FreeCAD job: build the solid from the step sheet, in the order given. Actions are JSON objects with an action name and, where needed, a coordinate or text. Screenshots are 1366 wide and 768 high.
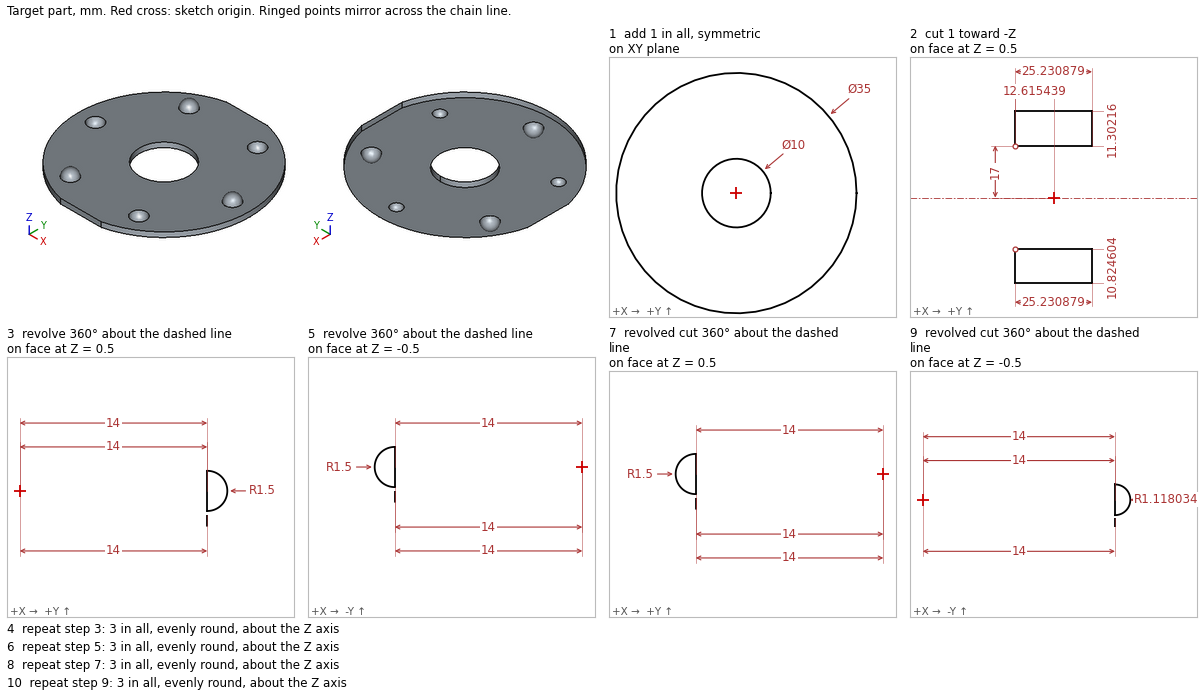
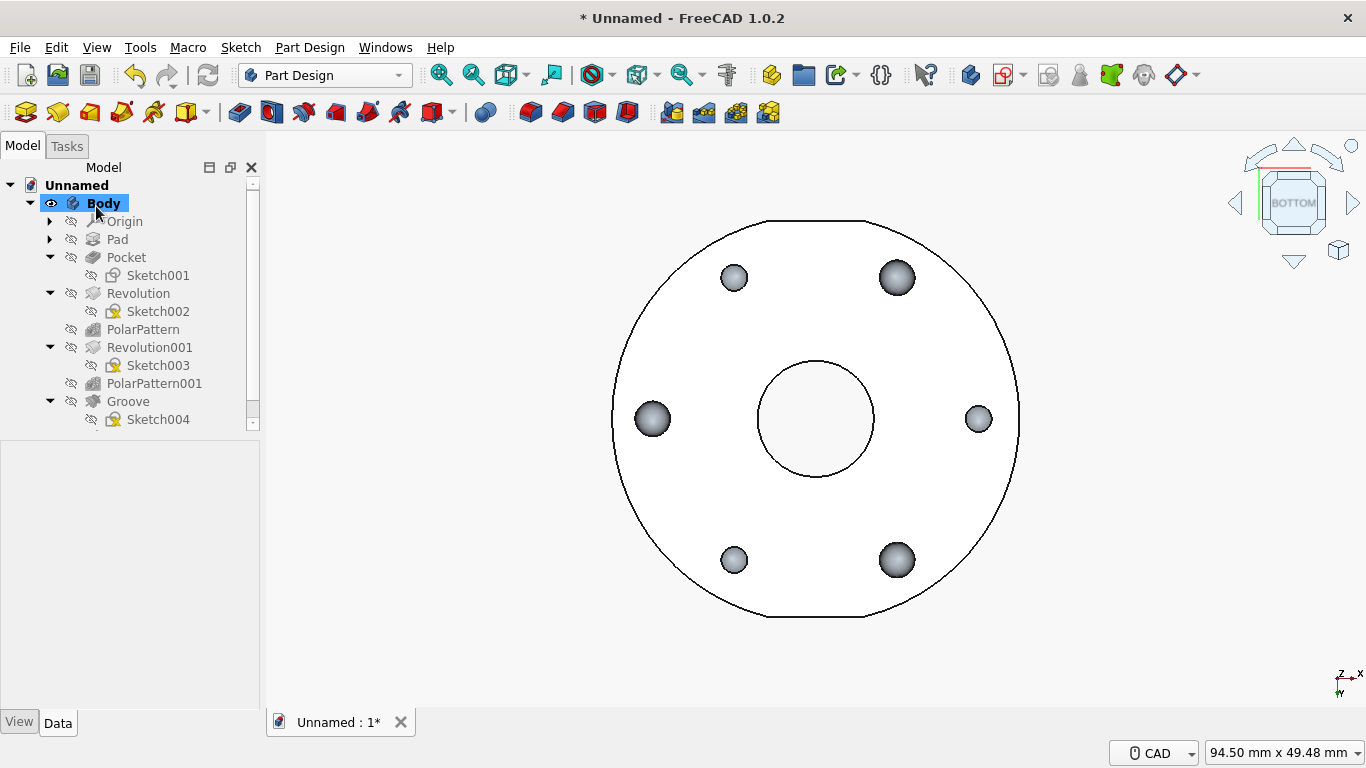
{"action": "left_click", "coordinate": [932, 361]}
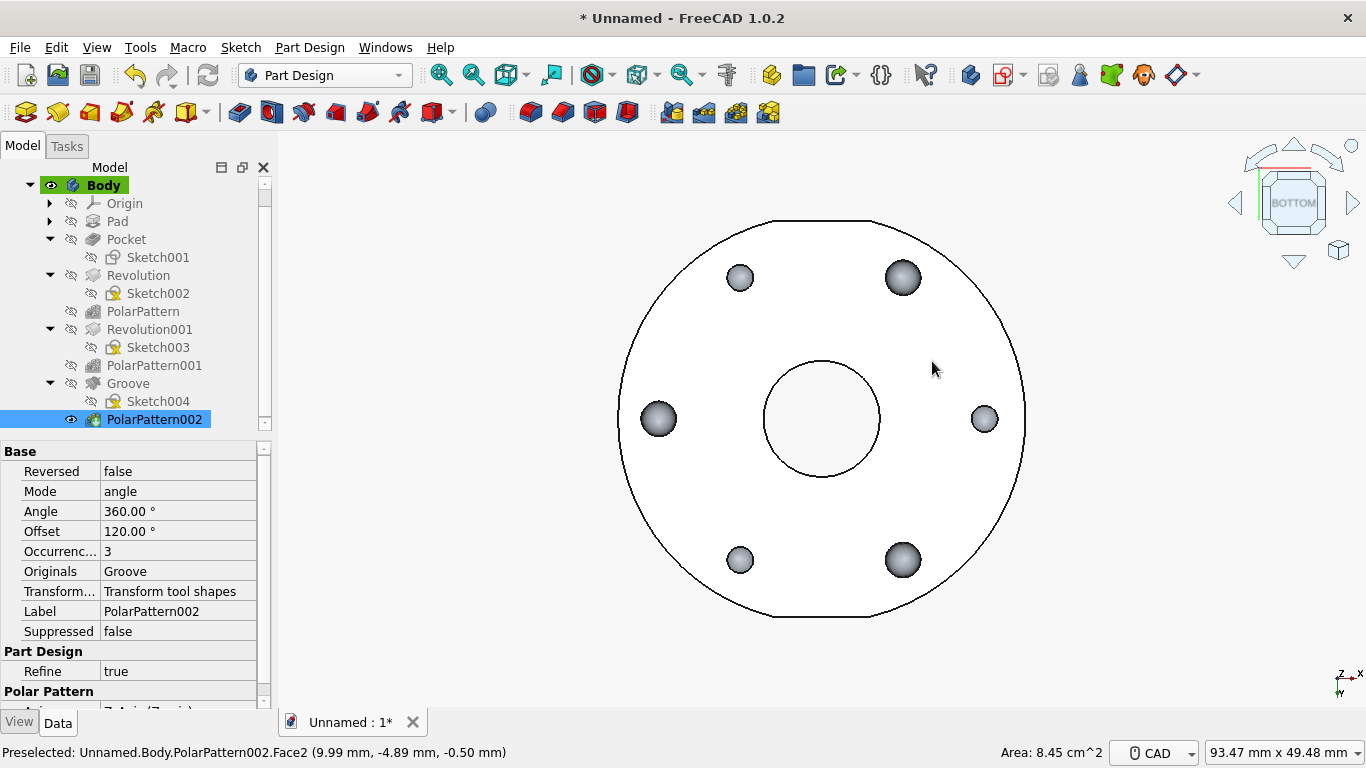
{"action": "left_click", "coordinate": [1004, 76]}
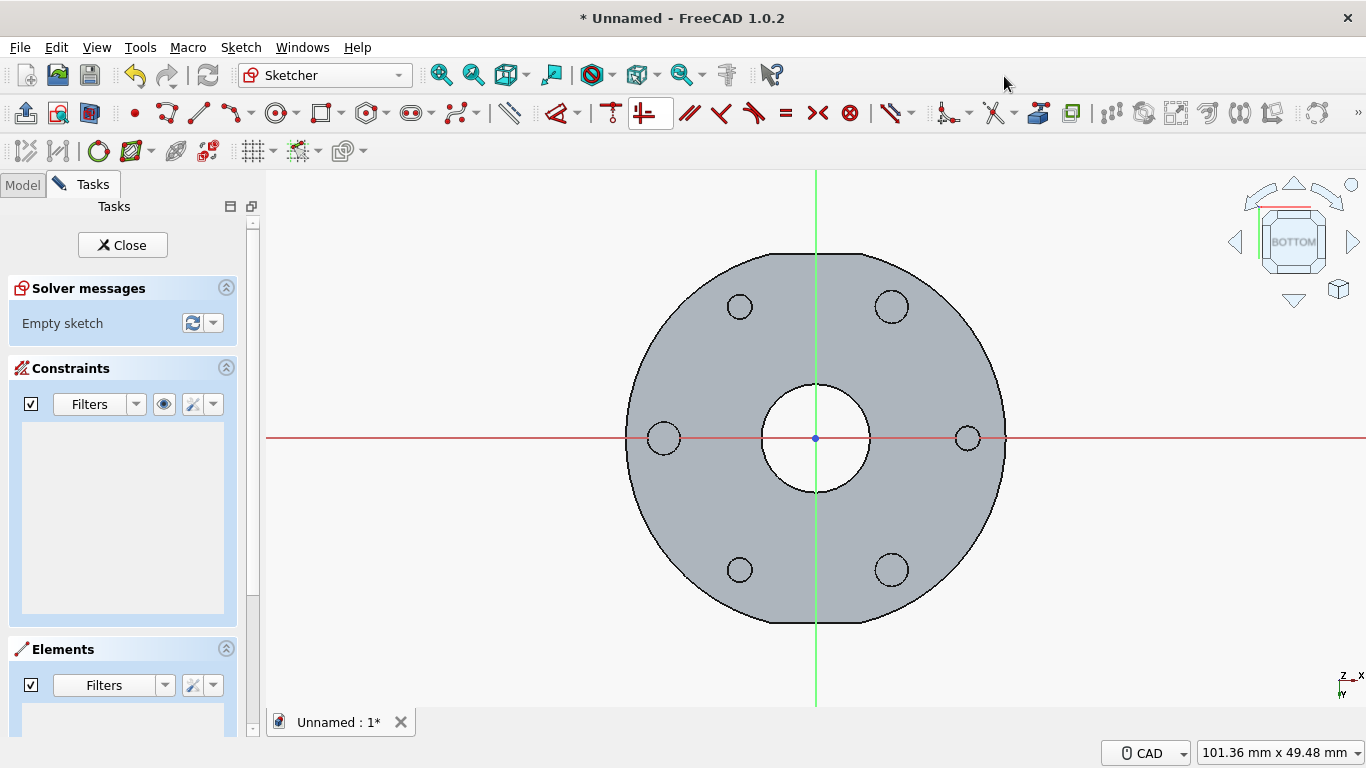
{"action": "left_click", "coordinate": [90, 114]}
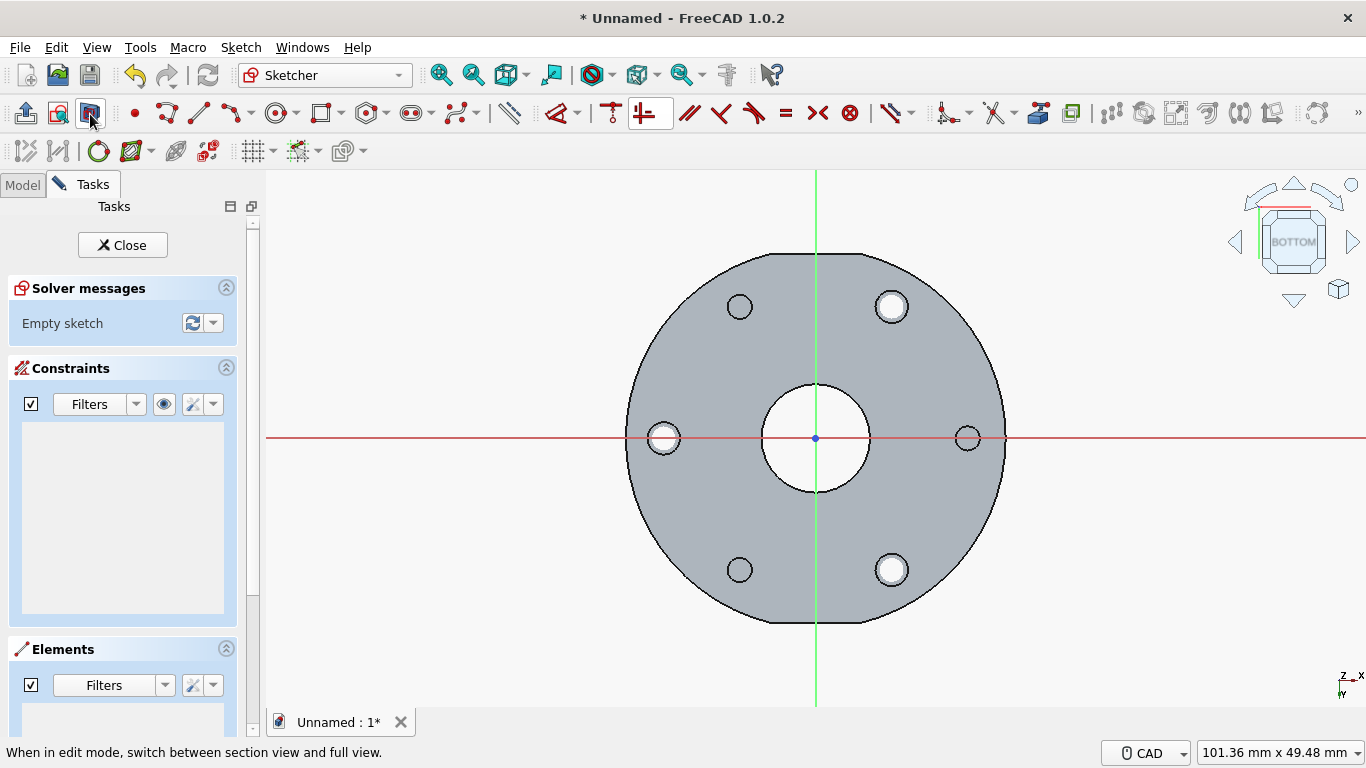
{"action": "scroll", "coordinate": [996, 444], "scroll_direction": "up", "scroll_amount": 12}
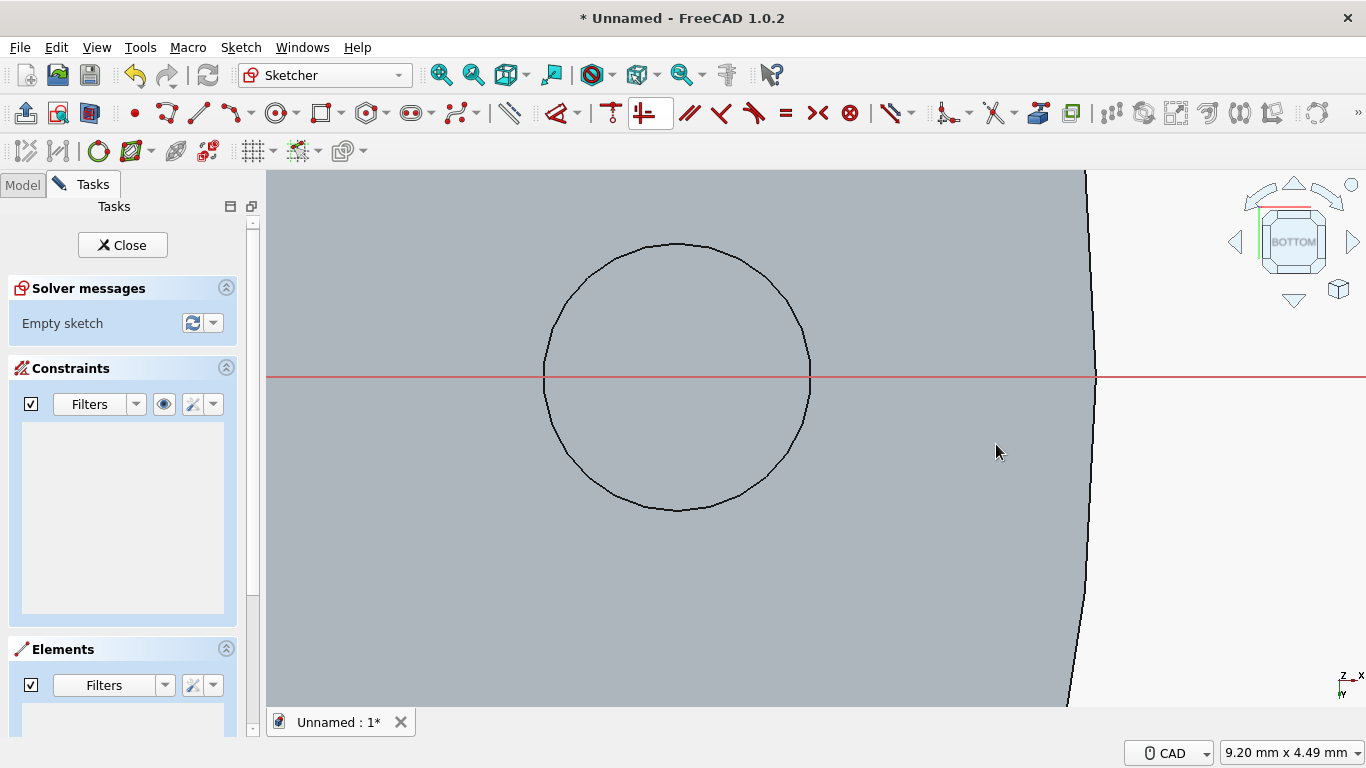
{"action": "key", "text": "g l"}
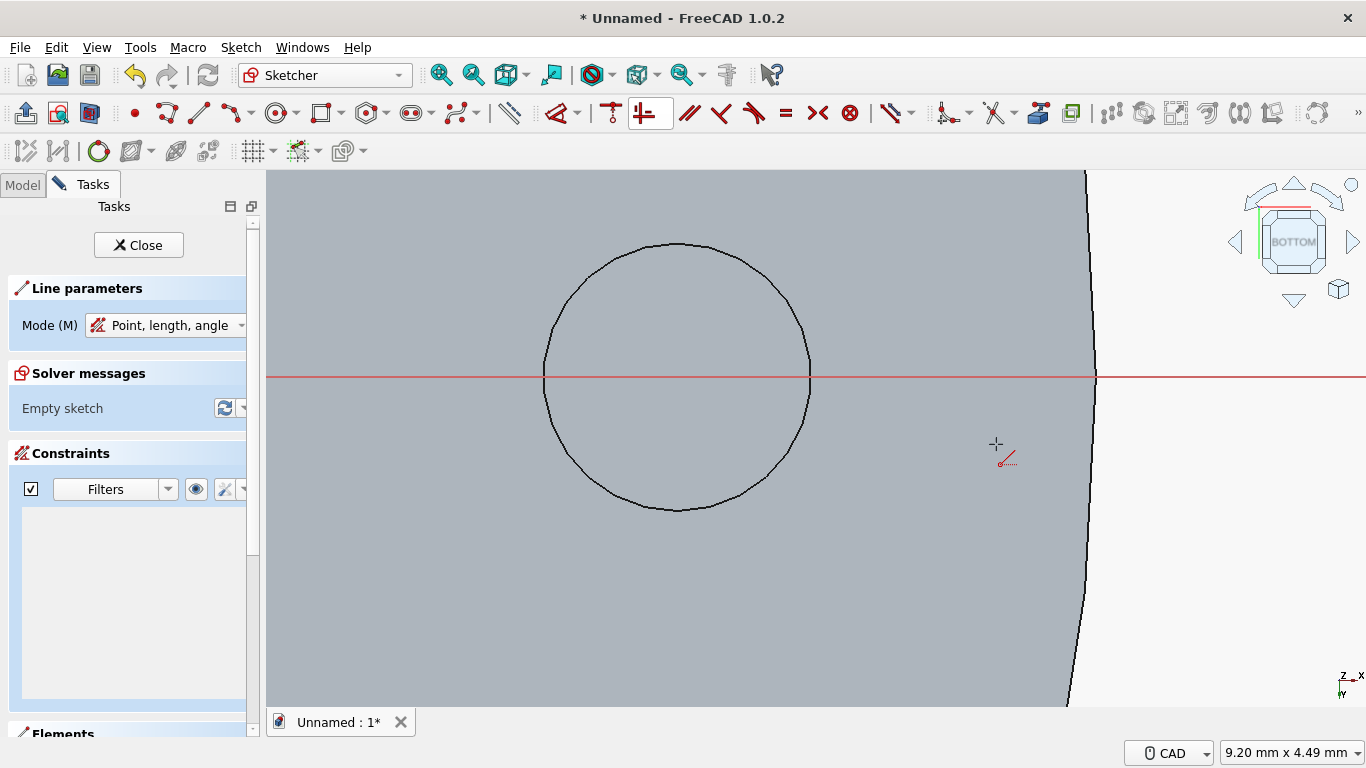
{"action": "left_click", "coordinate": [677, 244]}
{"action": "left_click", "coordinate": [677, 511]}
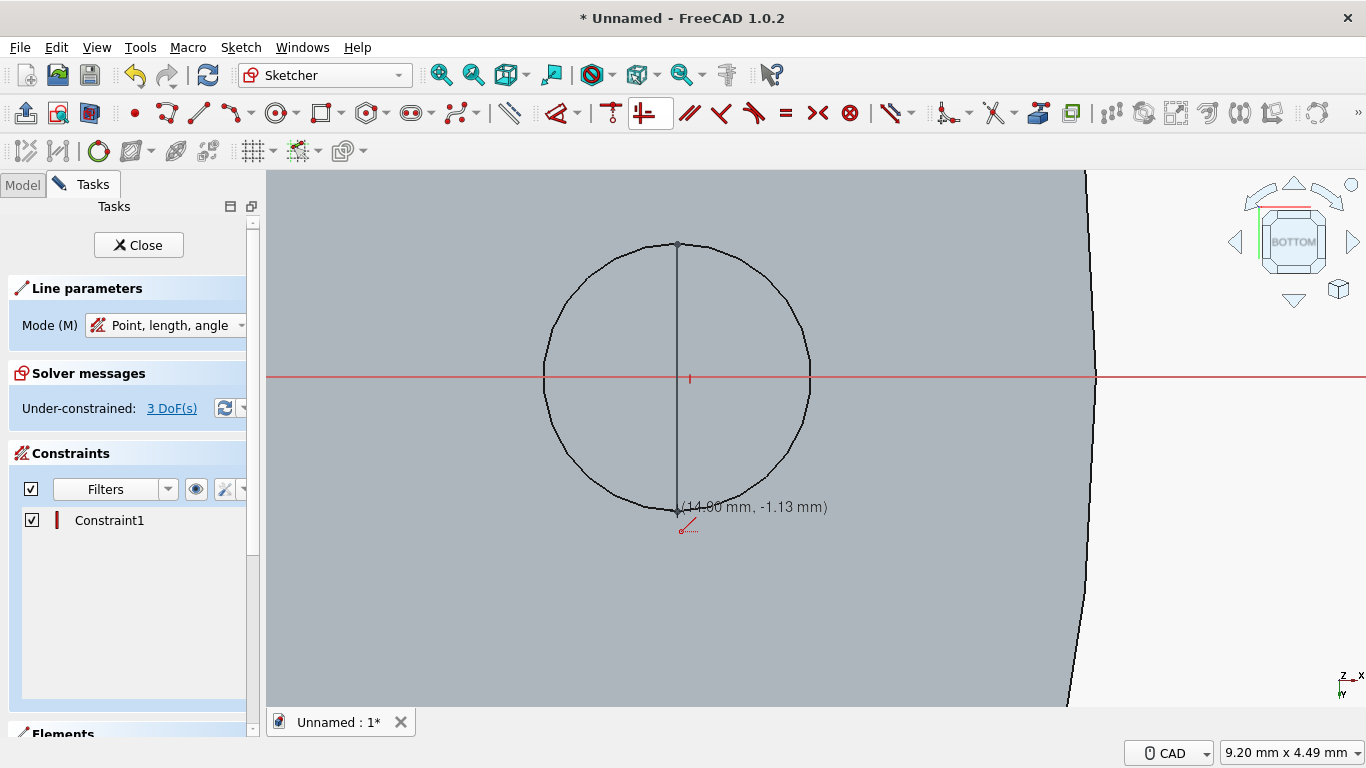
{"action": "key", "text": "g 3 a"}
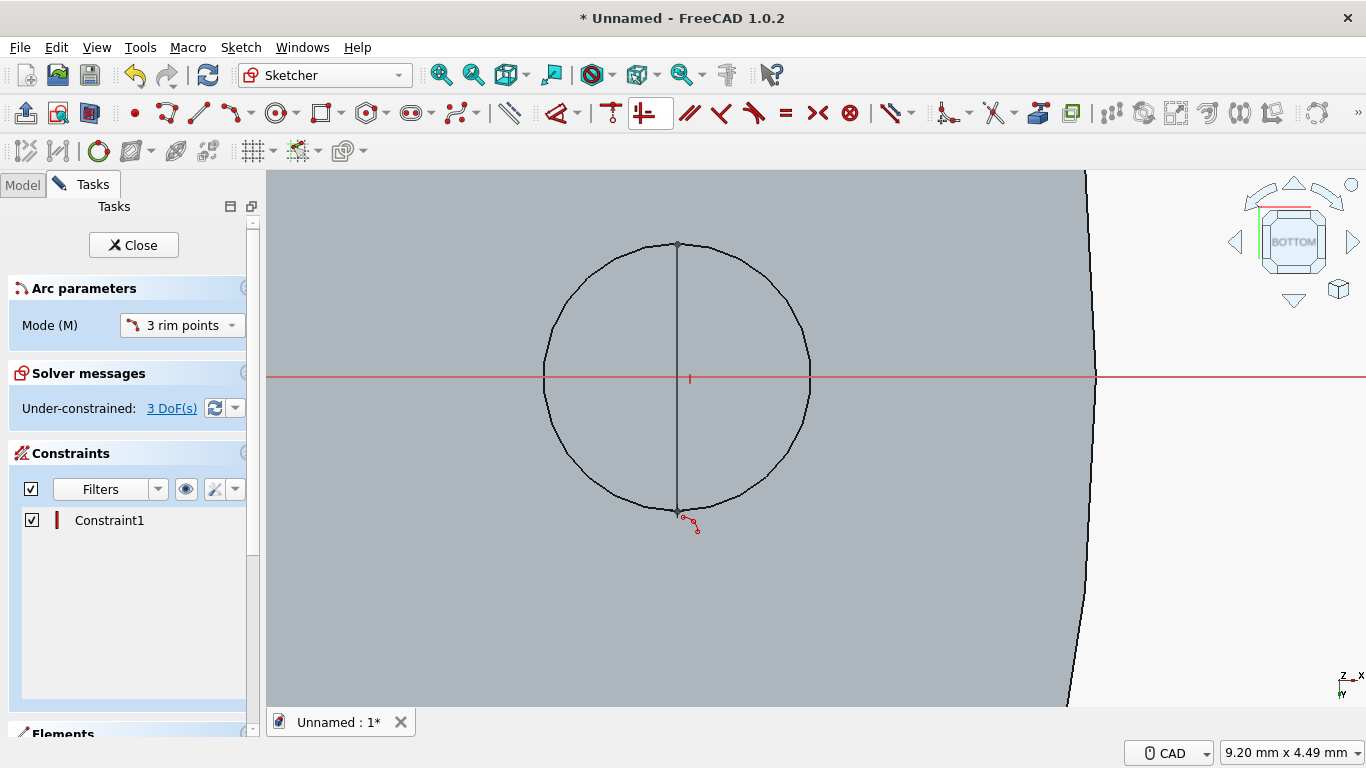
{"action": "left_click", "coordinate": [677, 512]}
{"action": "left_click", "coordinate": [677, 245]}
{"action": "left_click", "coordinate": [804, 419]}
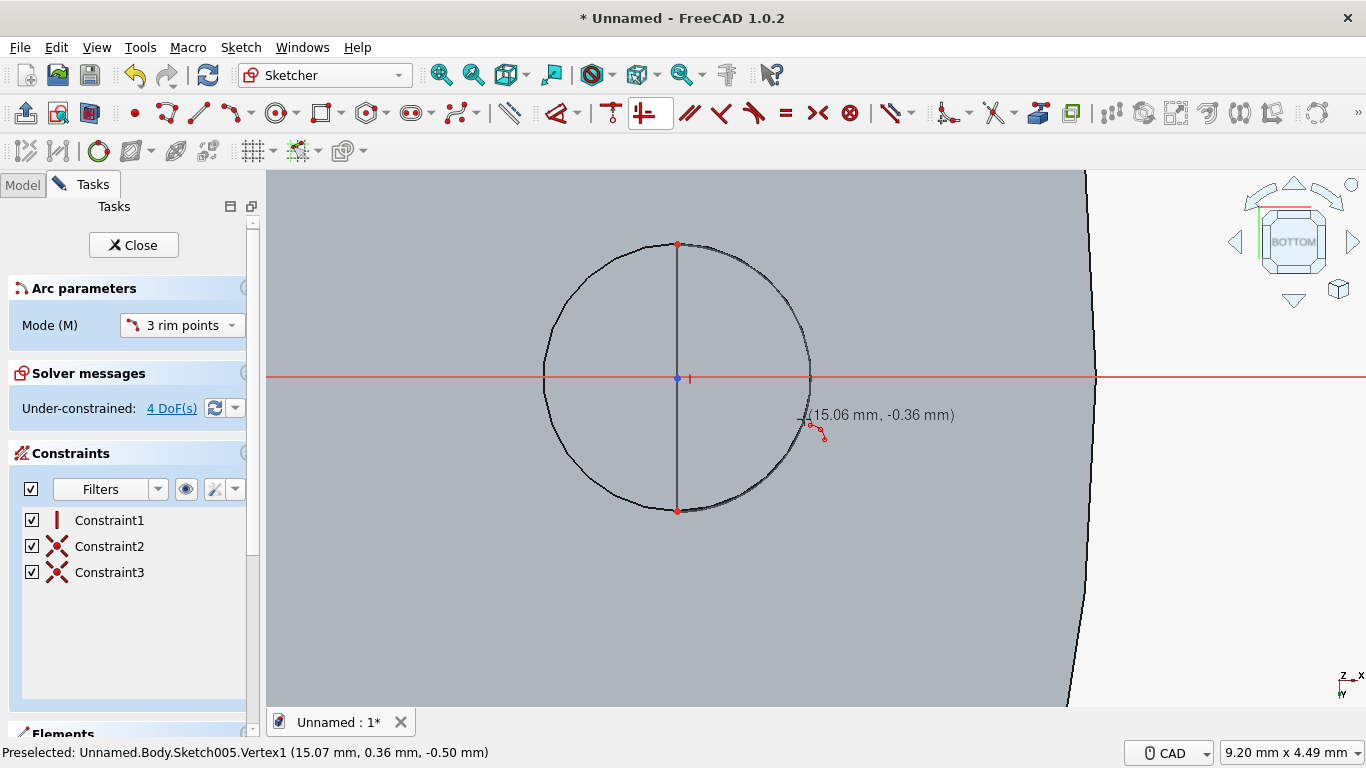
{"action": "key", "text": "g l"}